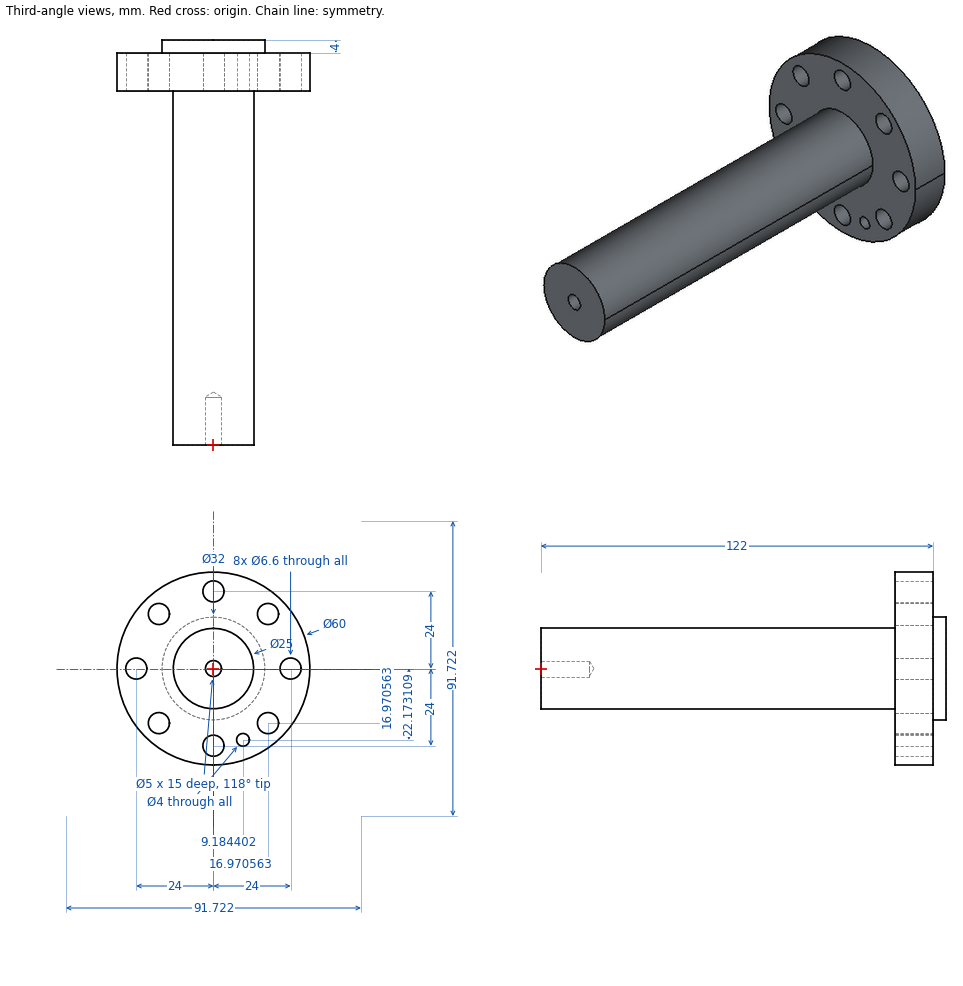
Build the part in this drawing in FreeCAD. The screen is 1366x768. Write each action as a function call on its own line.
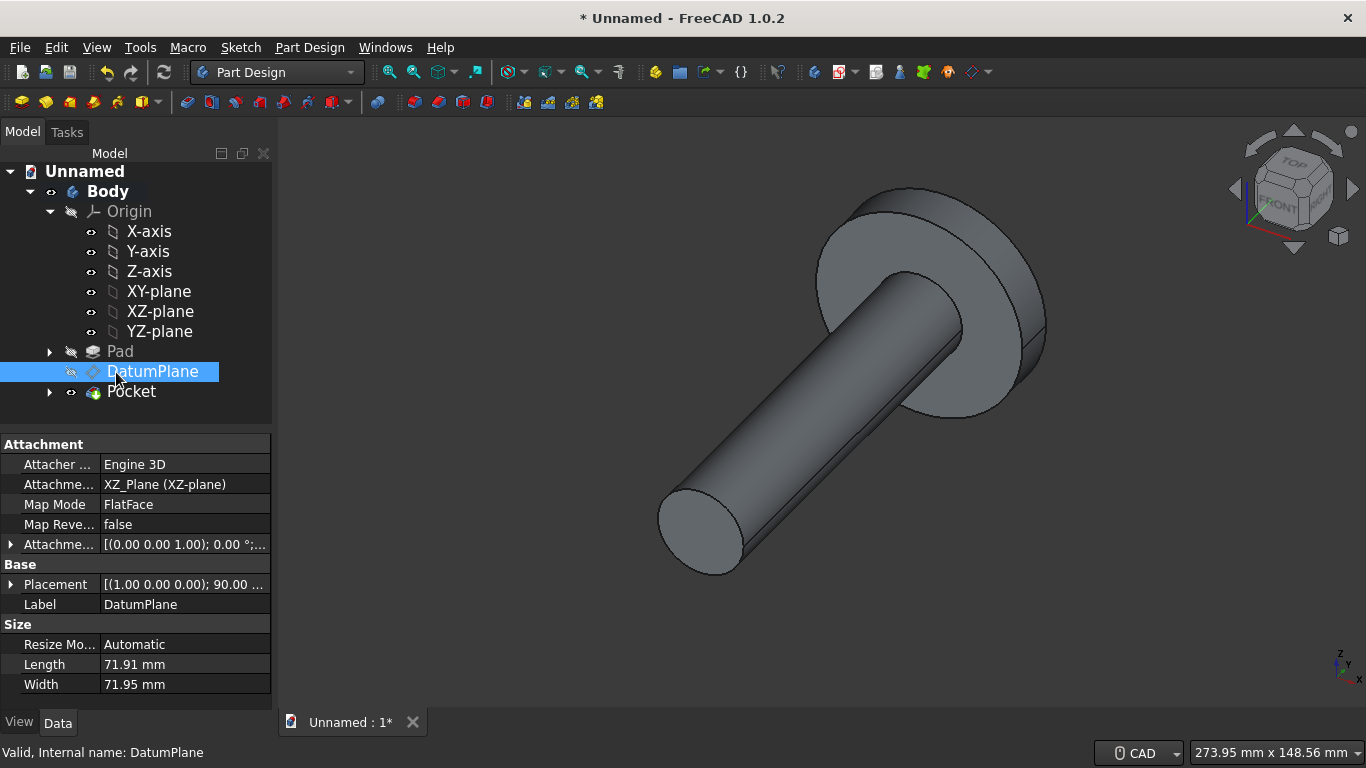
click(890, 249)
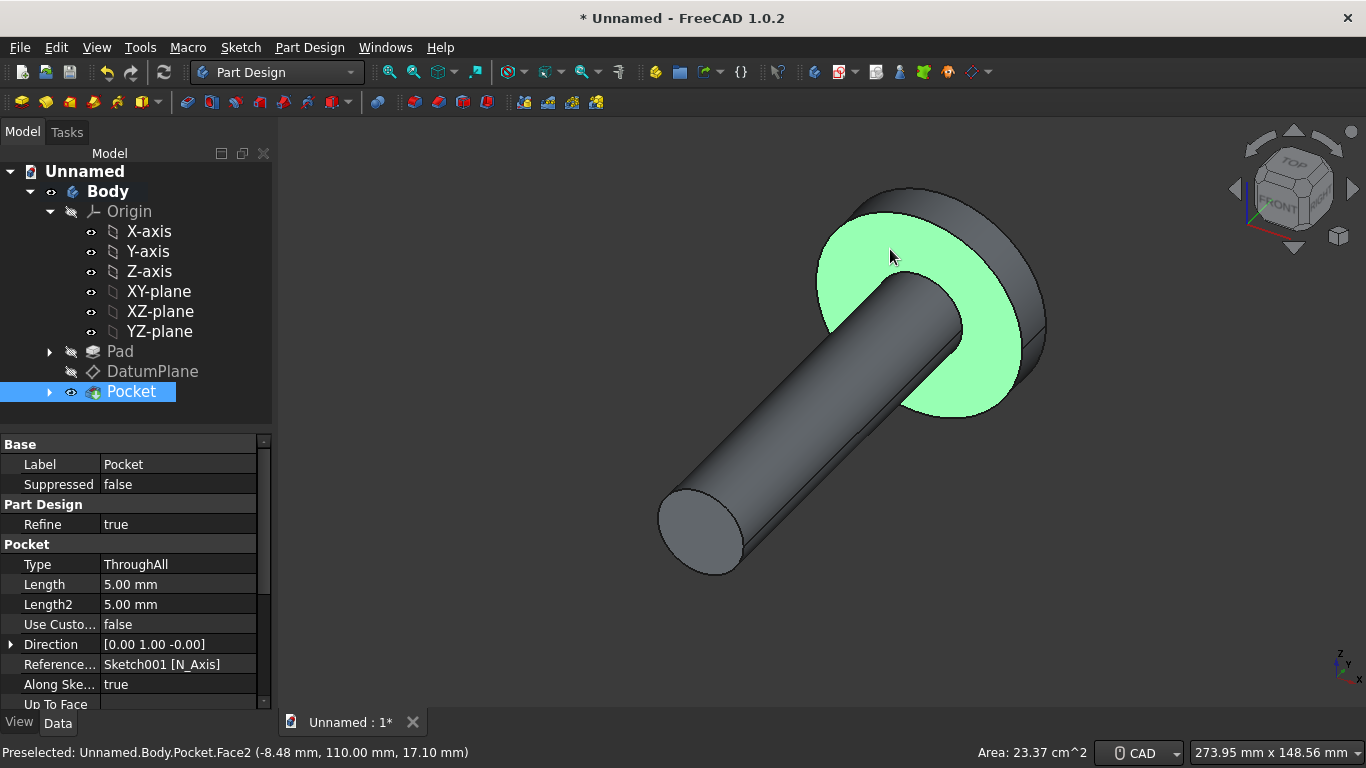
click(840, 72)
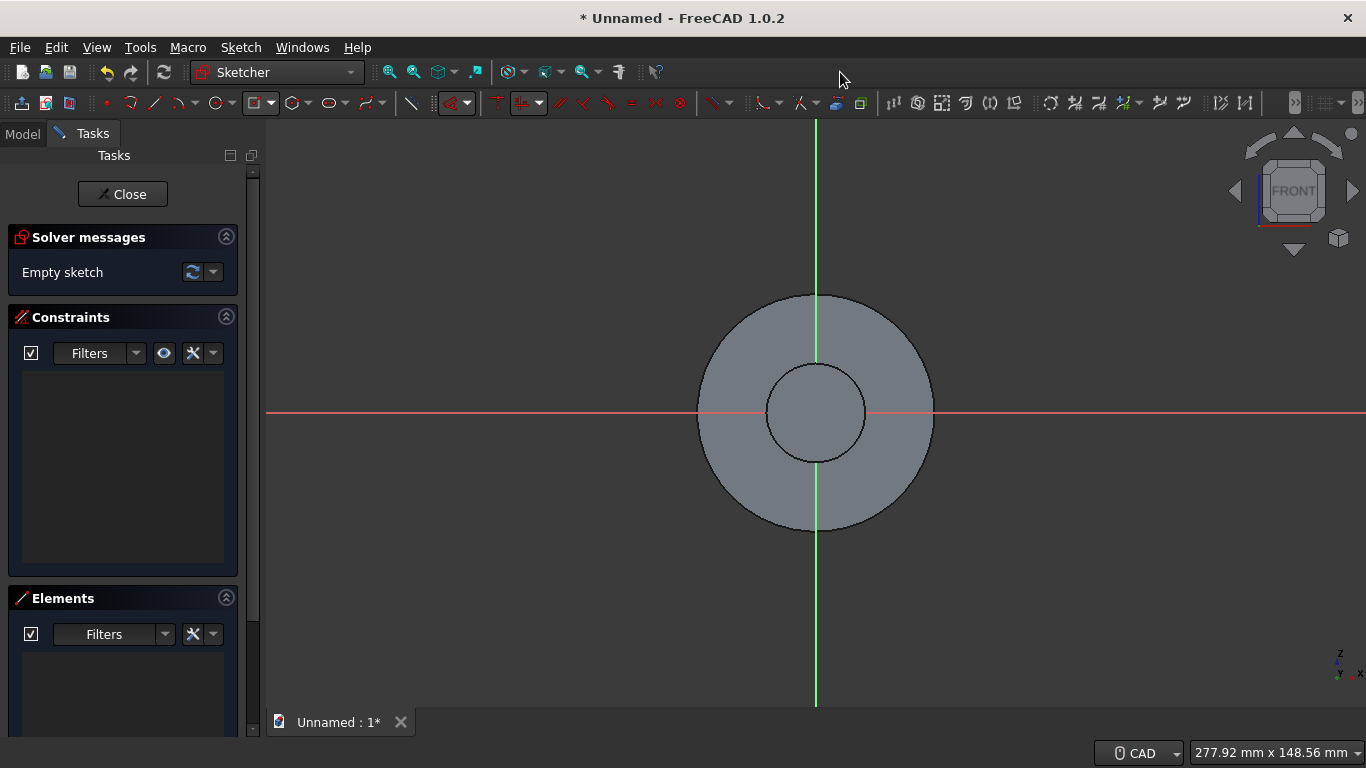
click(70, 104)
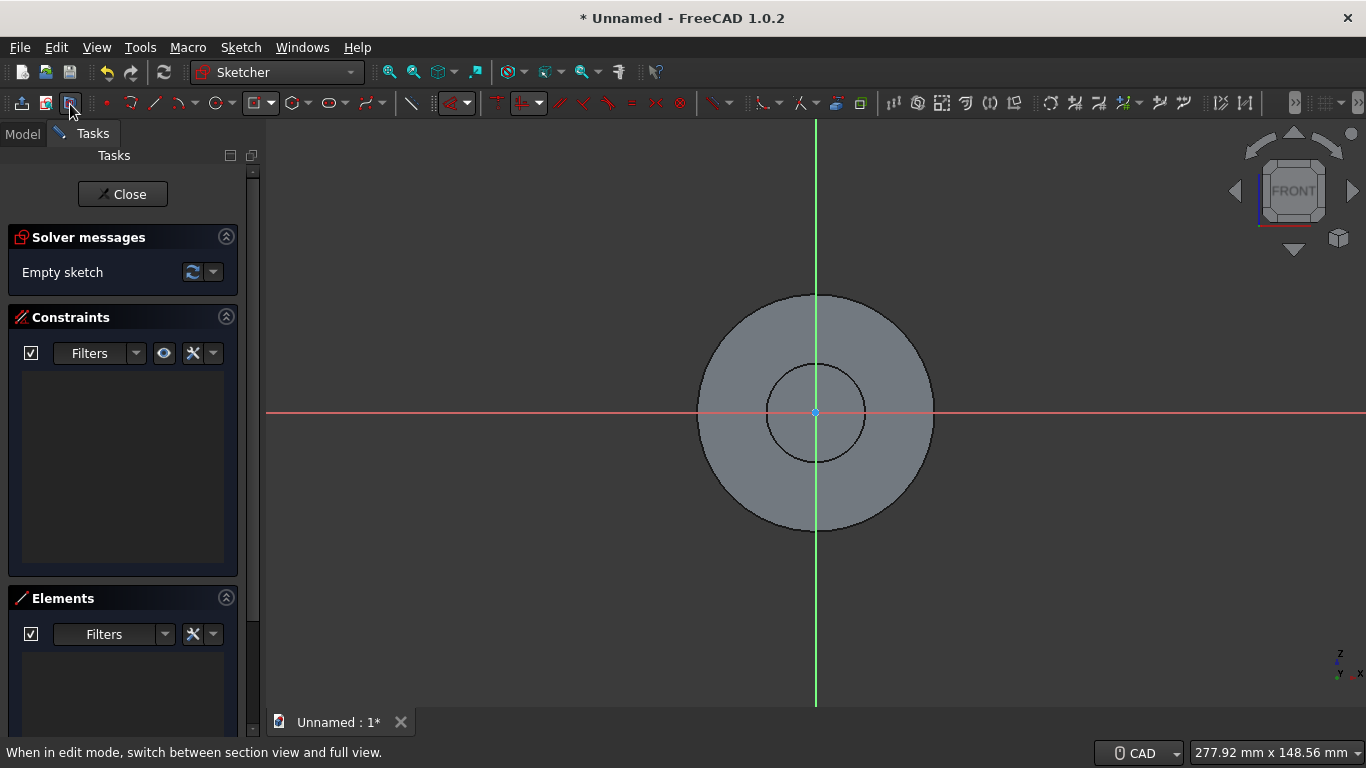
scroll(899, 413, up, 3)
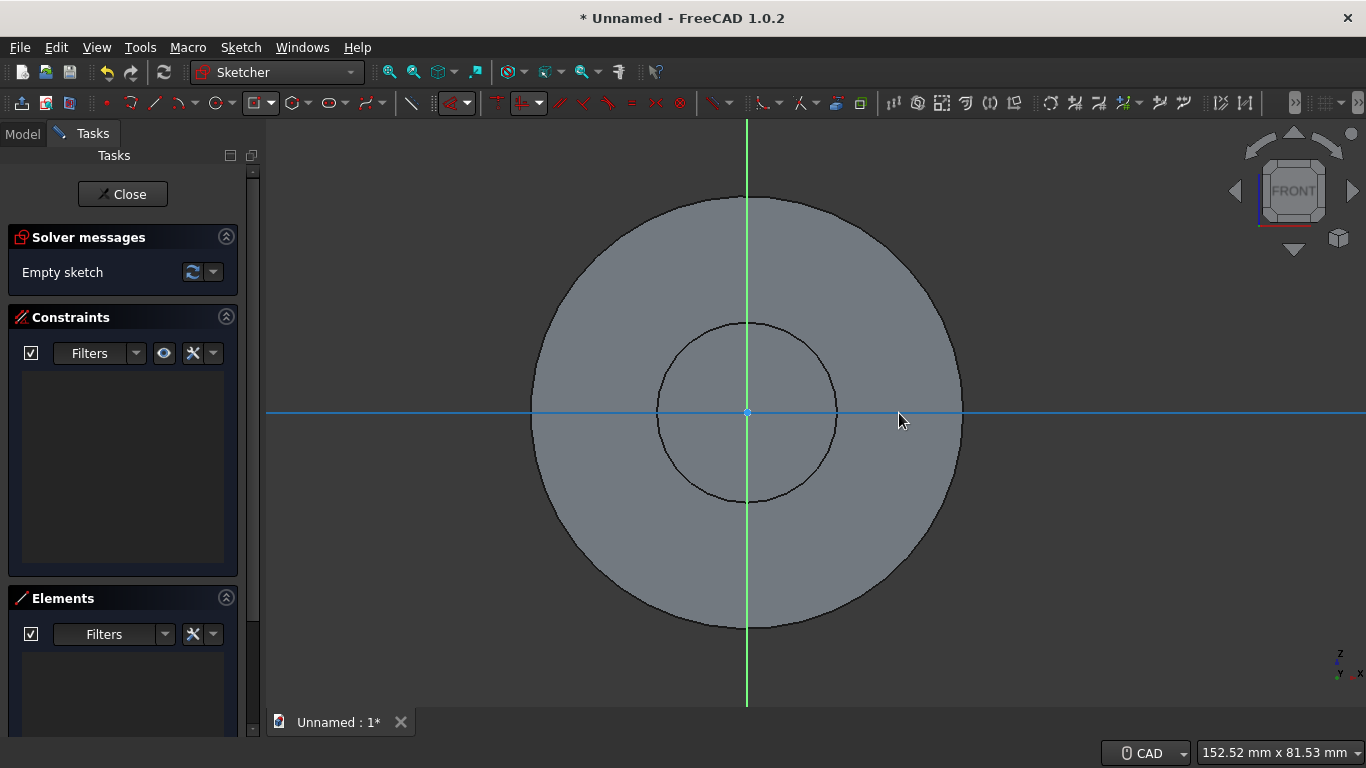
click(216, 104)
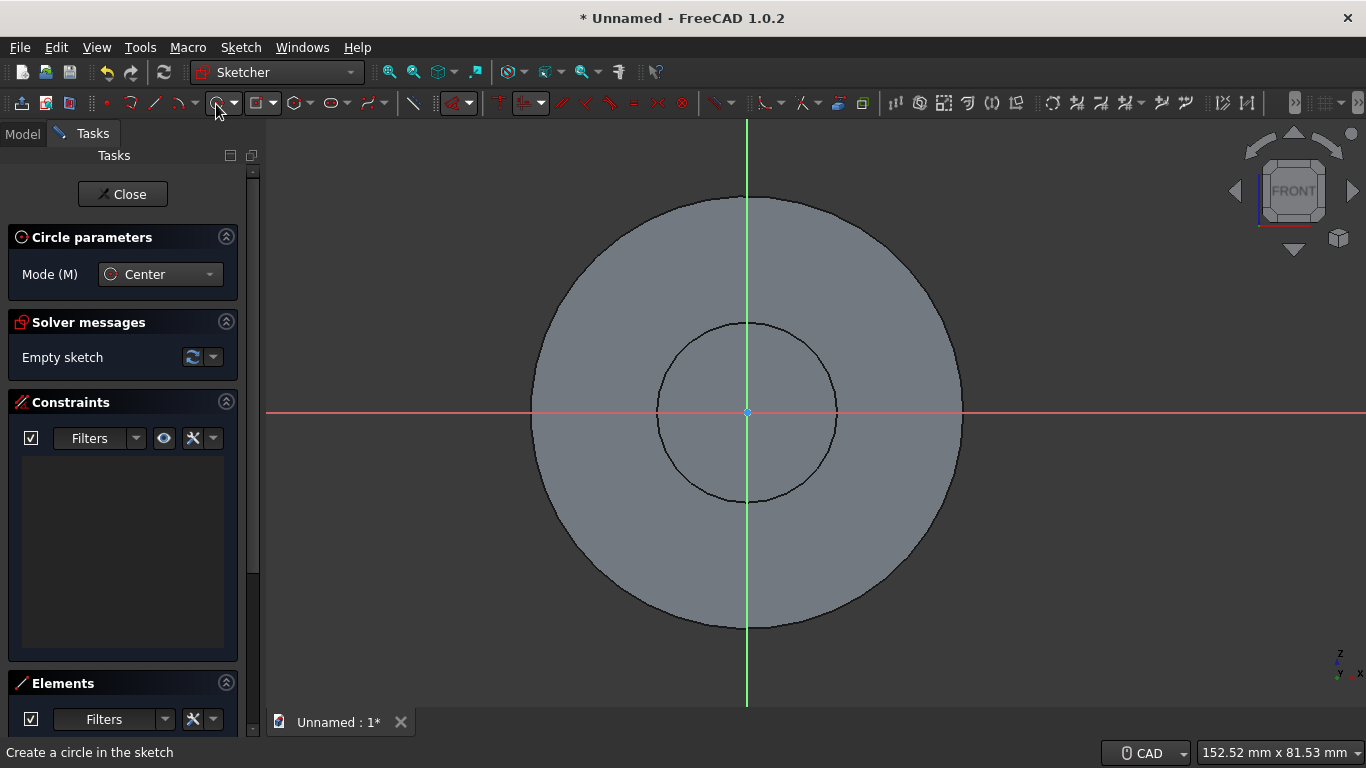
click(920, 413)
click(937, 396)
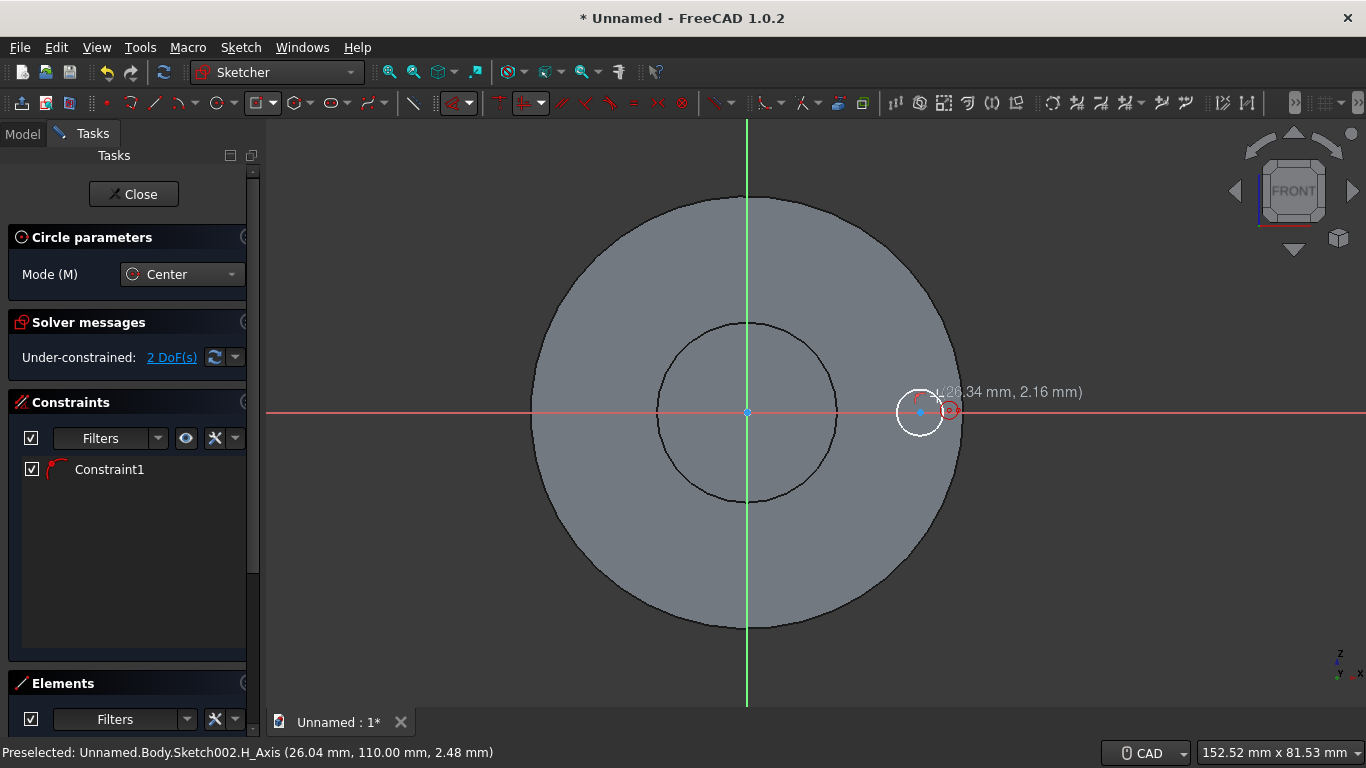
click(869, 535)
click(886, 518)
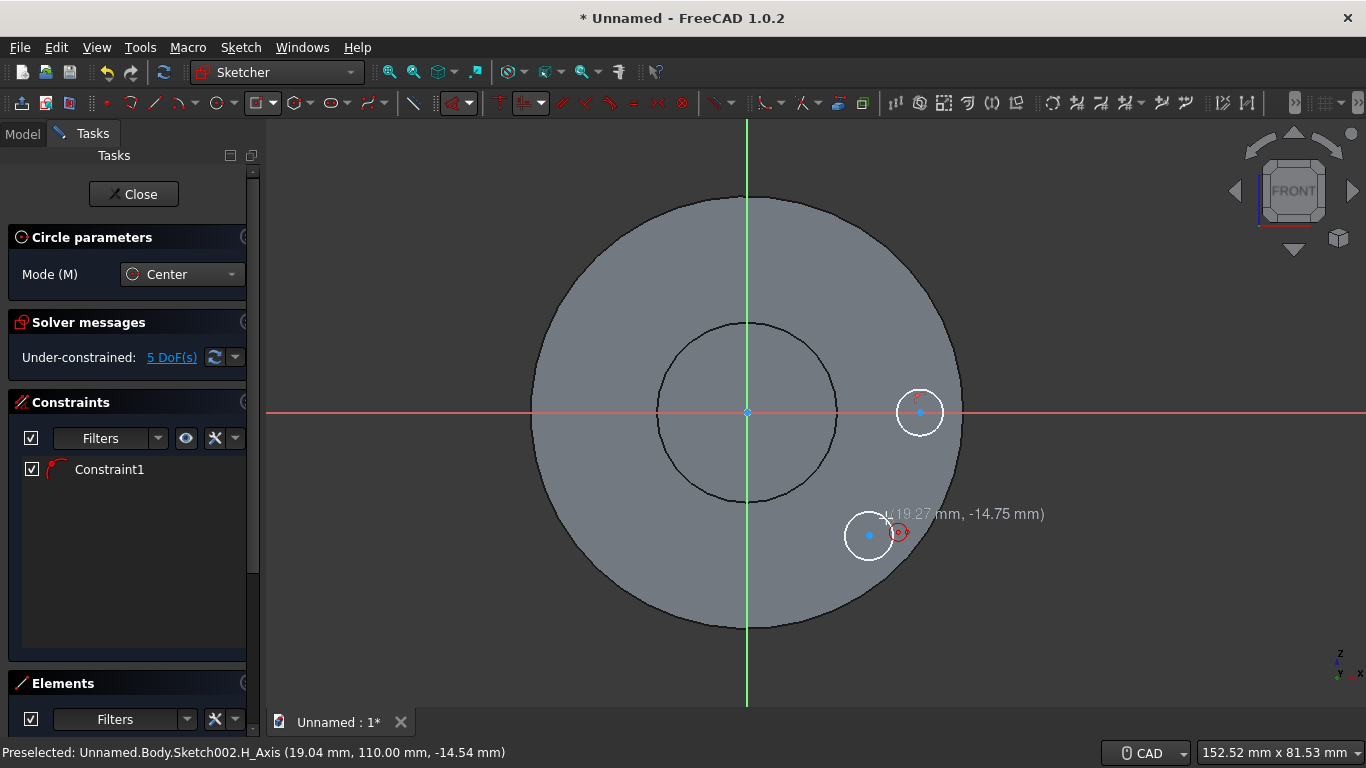
click(747, 586)
click(764, 569)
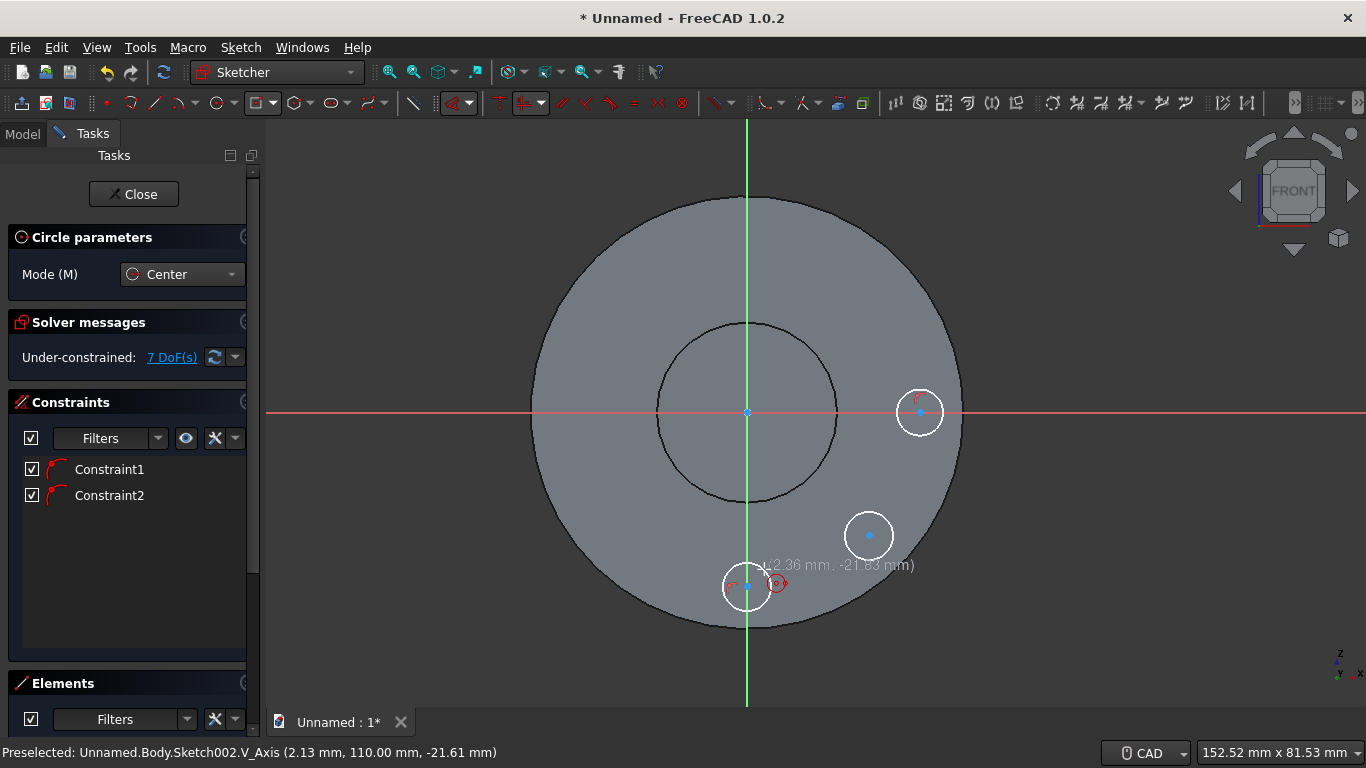
click(625, 535)
click(641, 518)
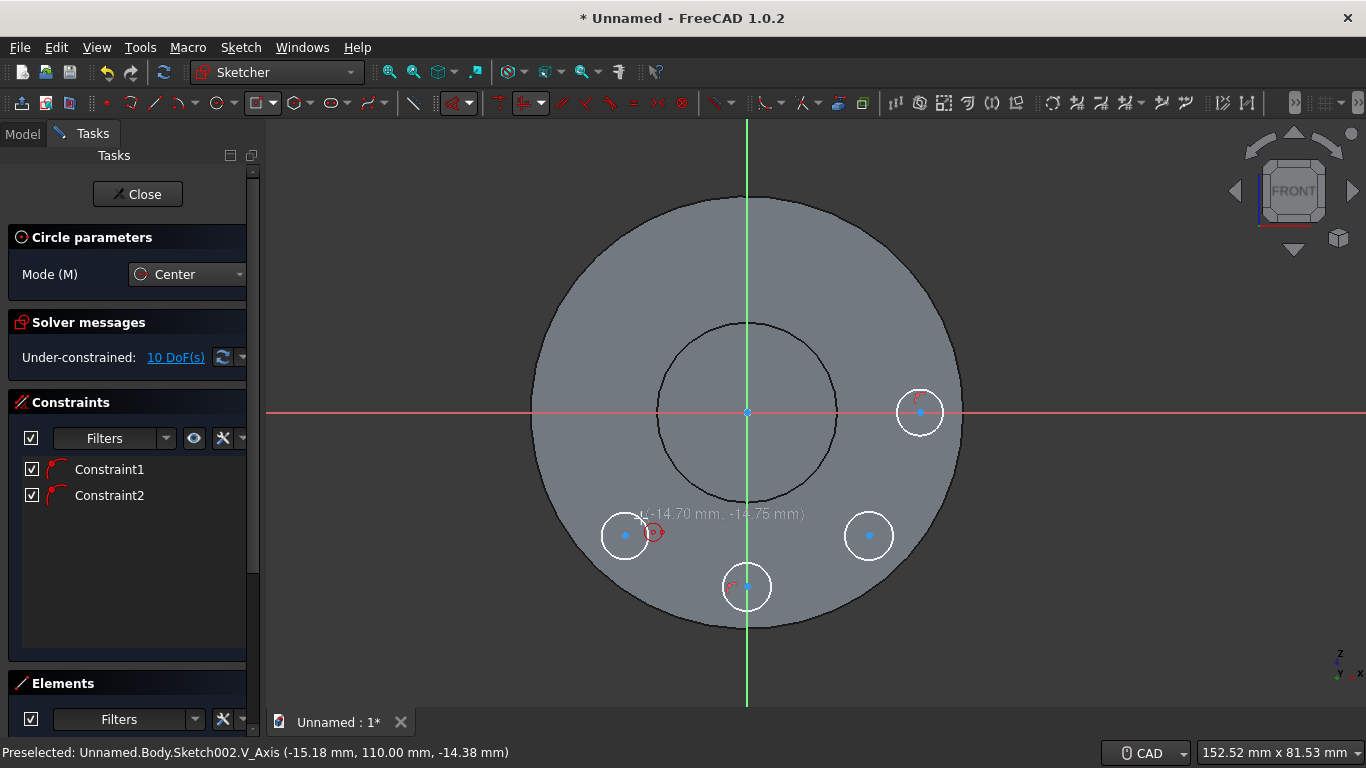
click(574, 413)
click(591, 396)